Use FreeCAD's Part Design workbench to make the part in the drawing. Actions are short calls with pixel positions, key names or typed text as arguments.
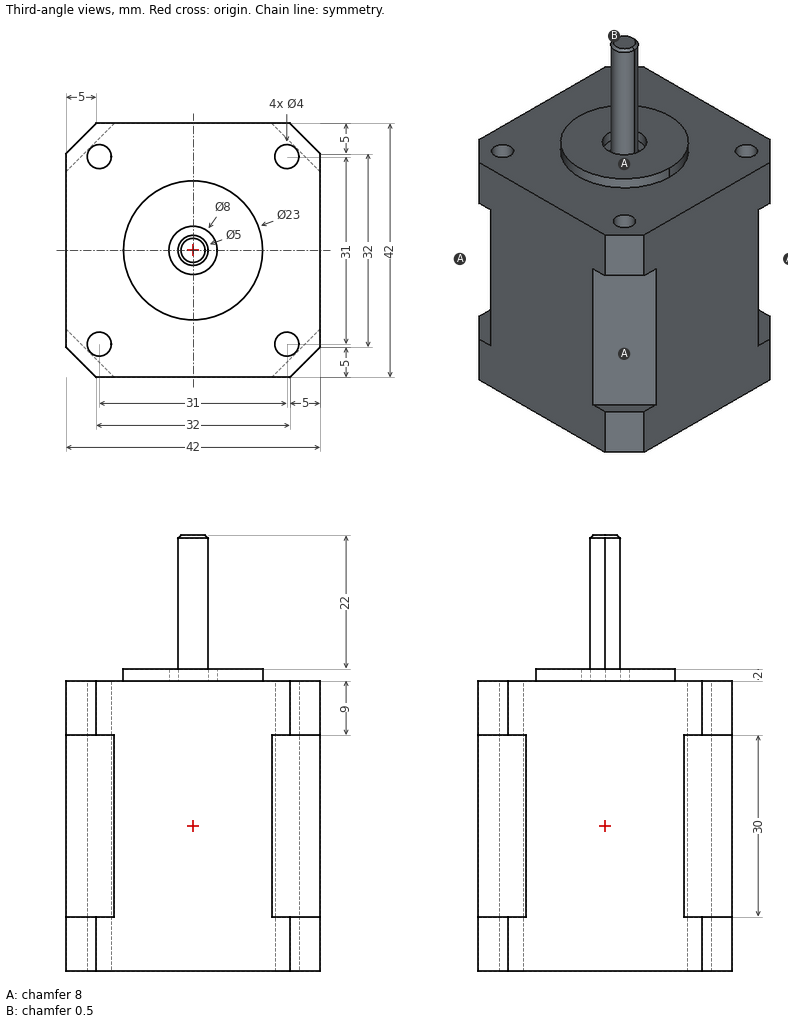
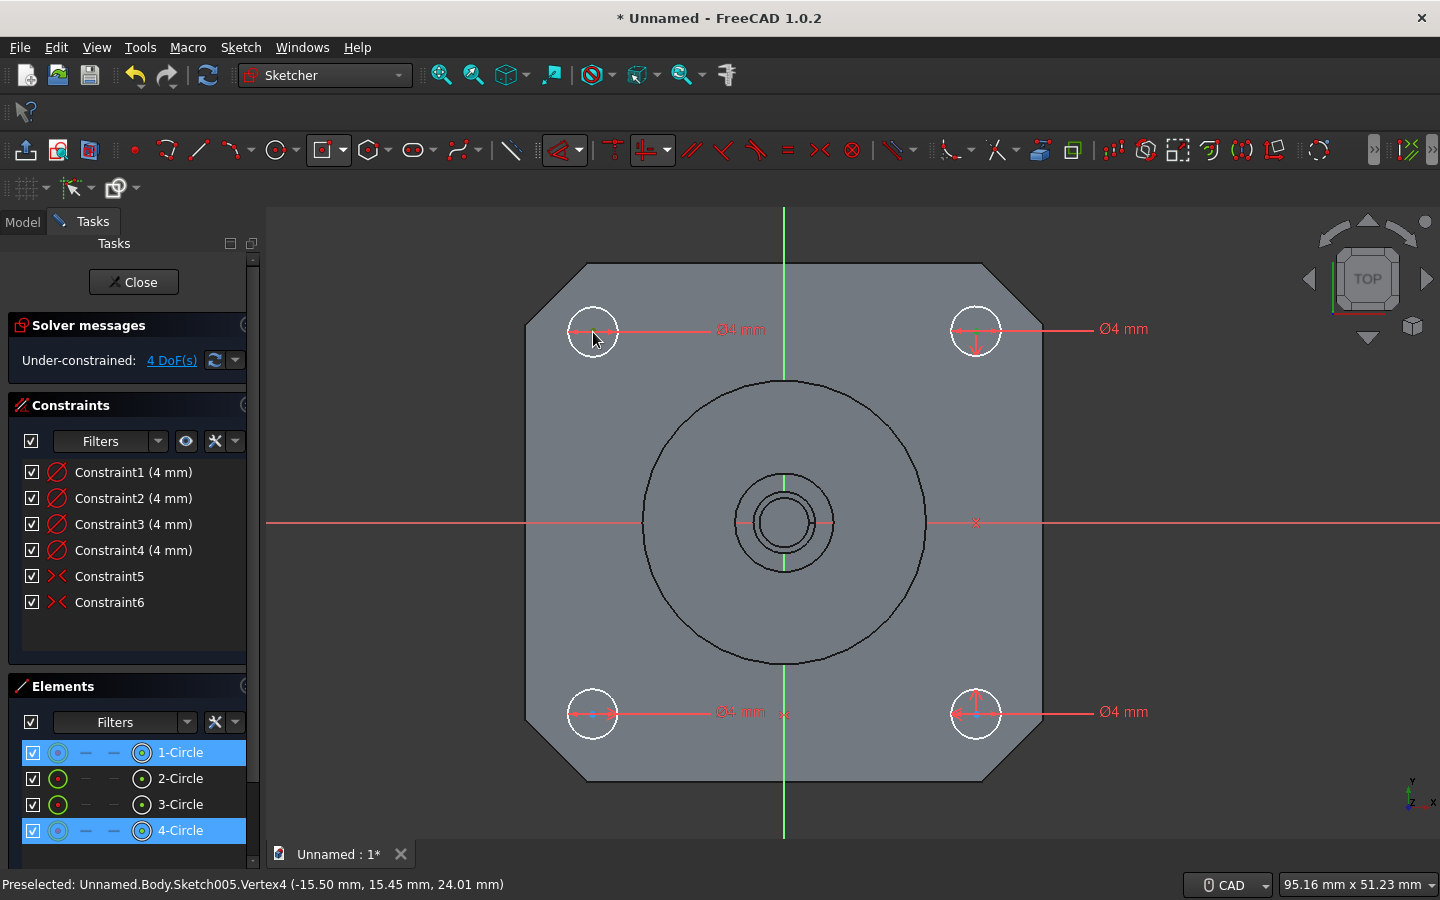
click(784, 770)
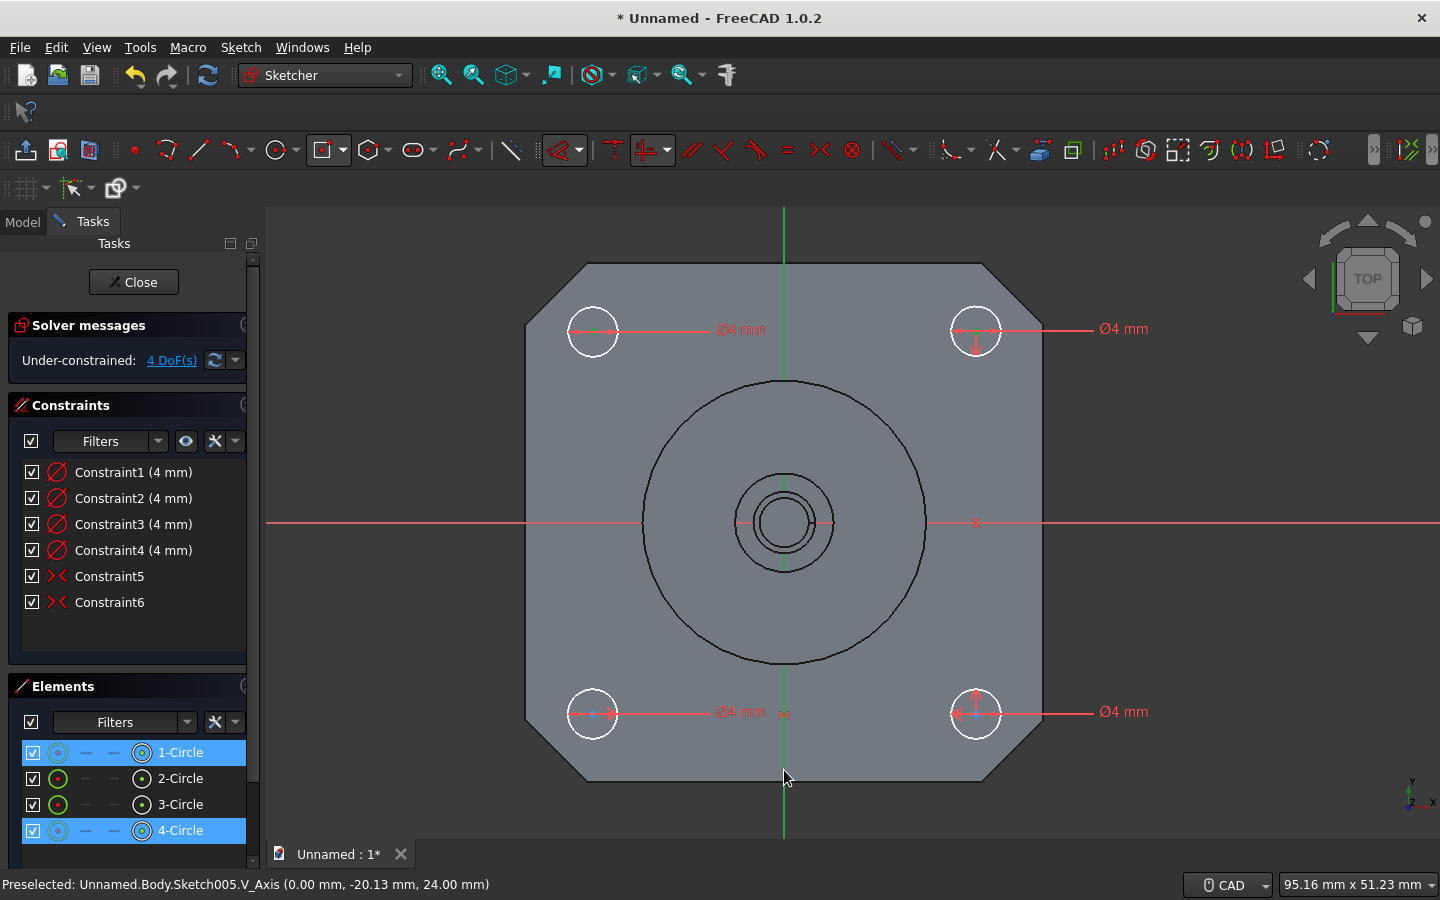
key(s)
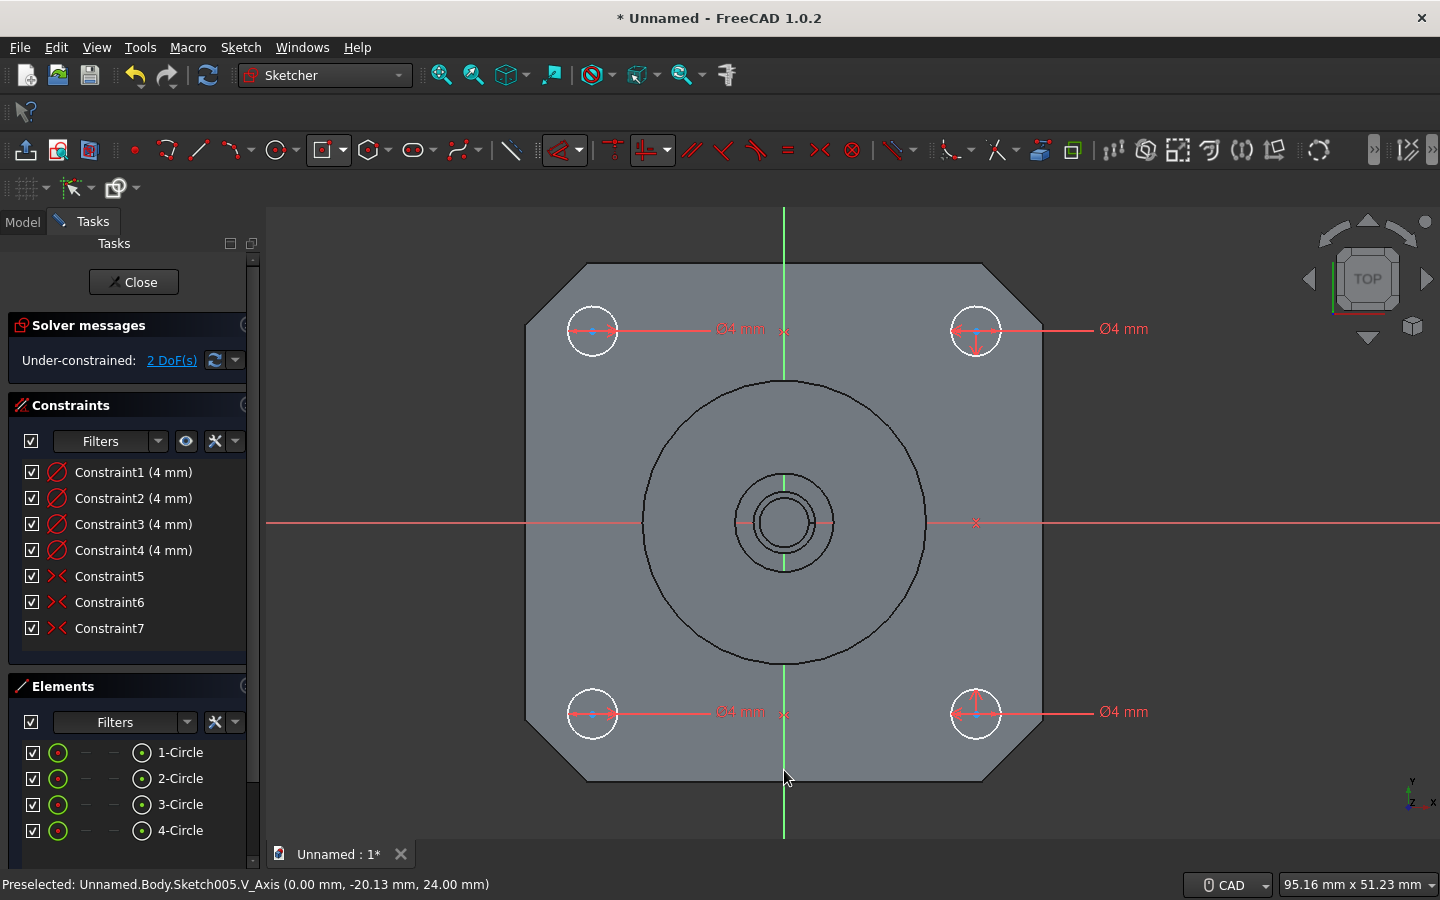
click(976, 331)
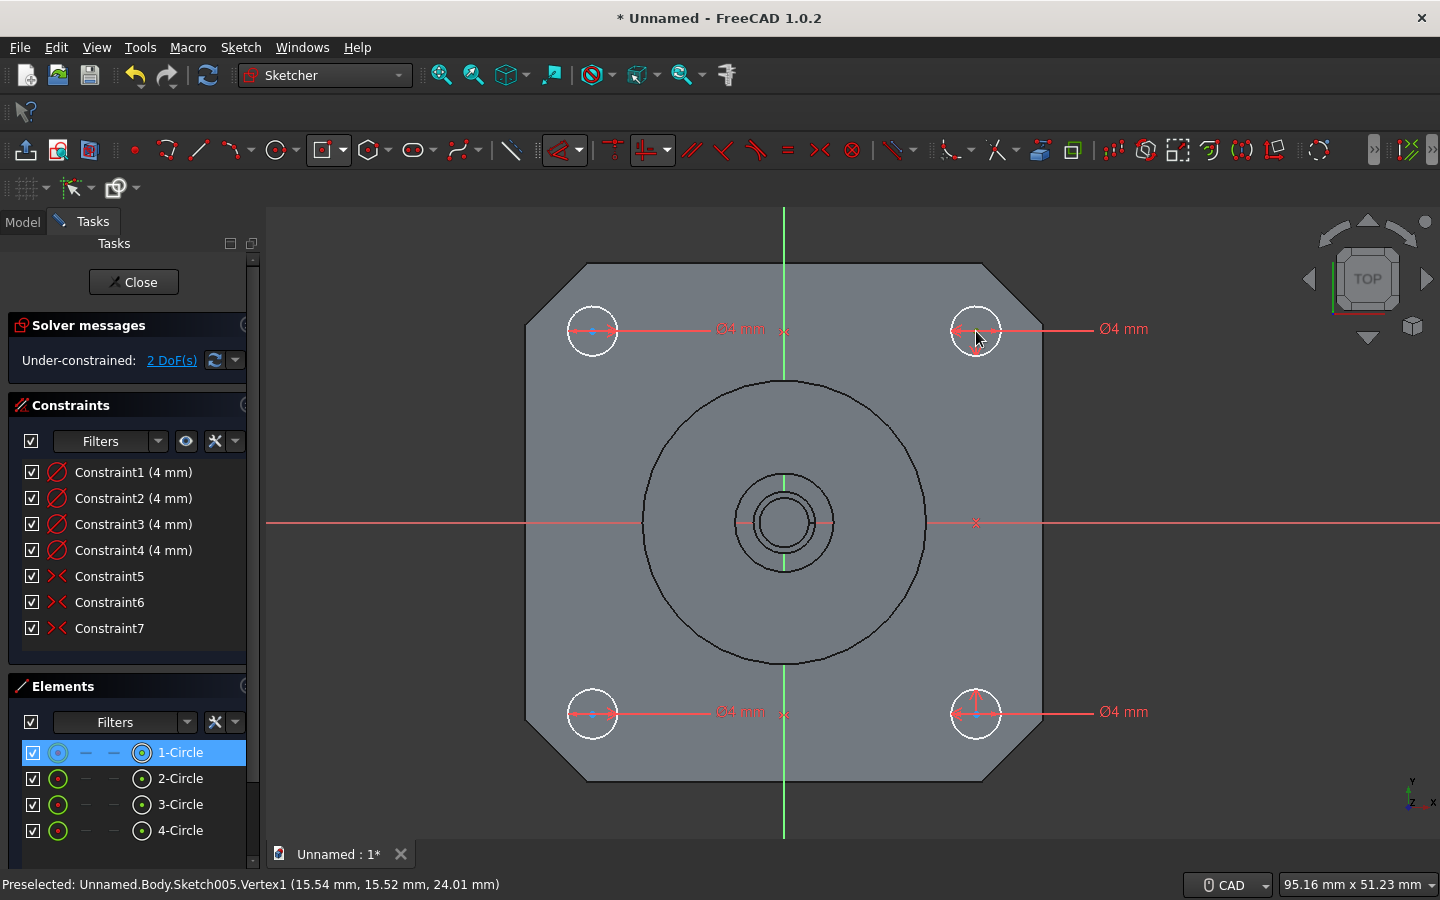
click(976, 714)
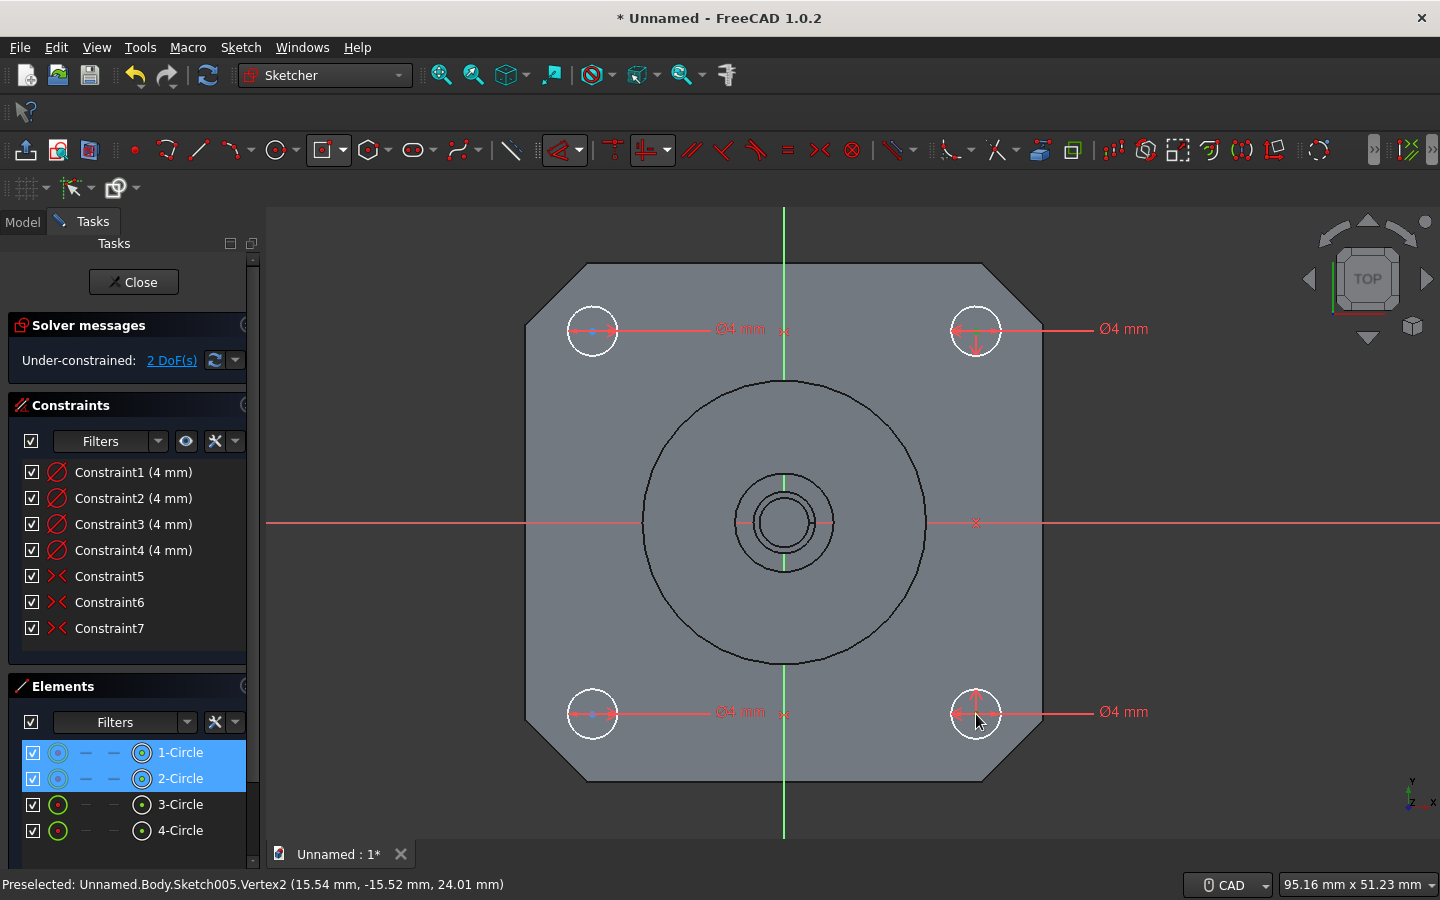
key(i)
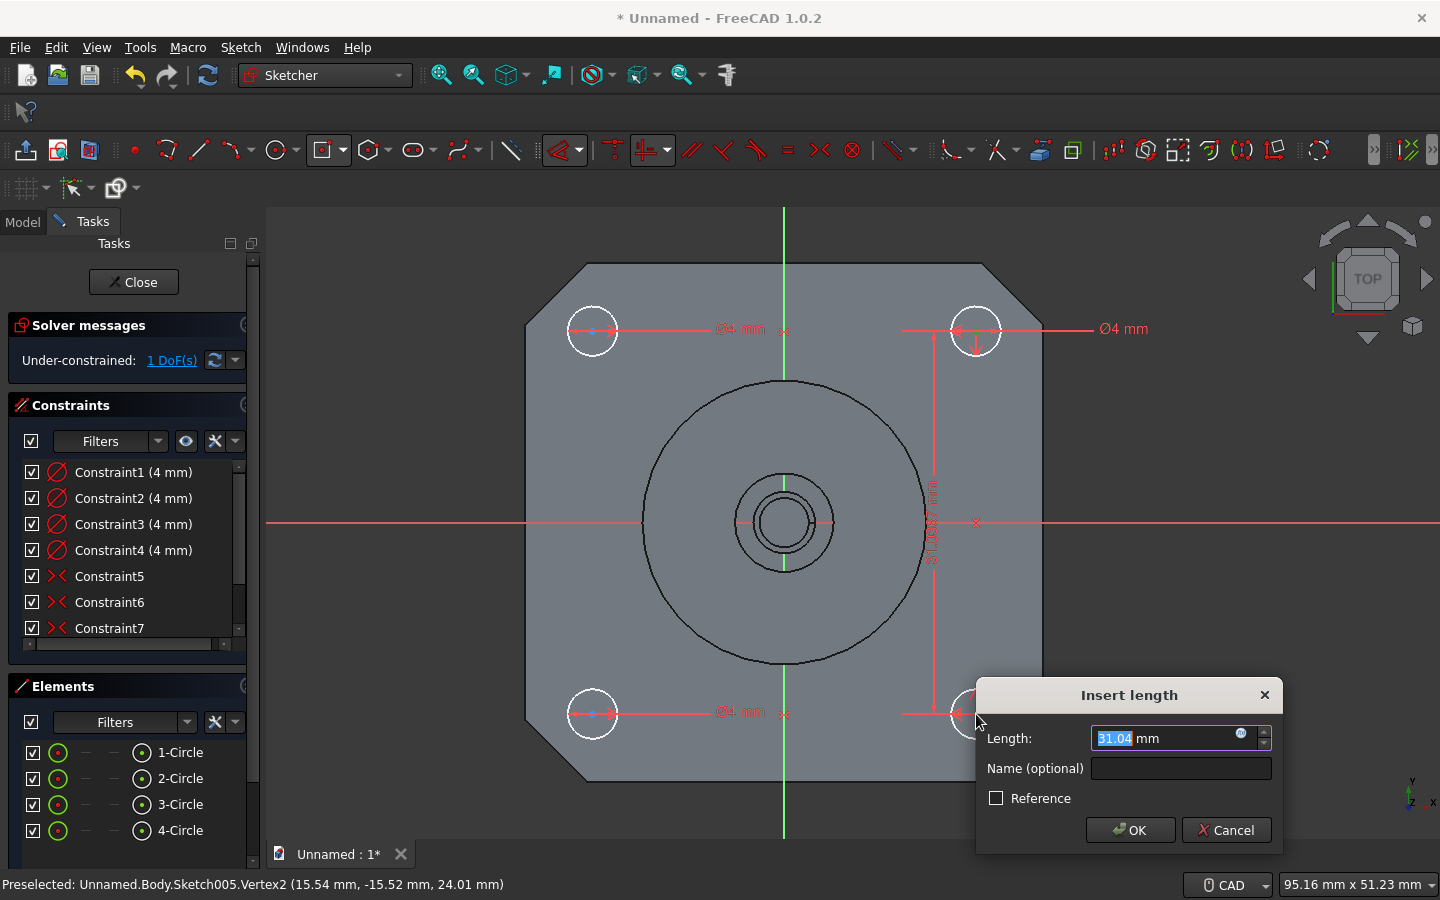
text(31)
key(Return)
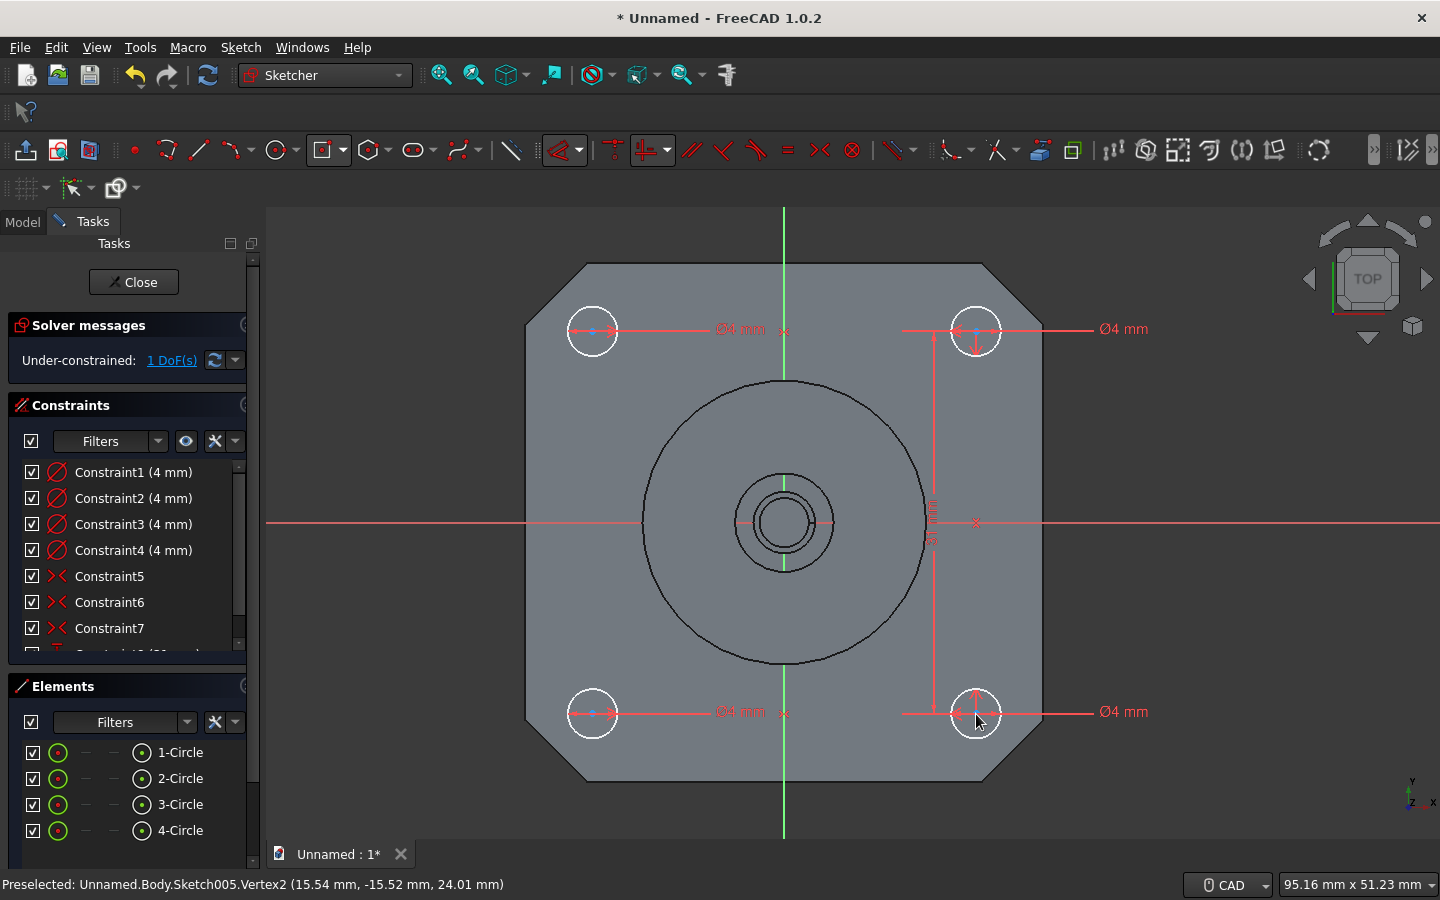
click(976, 714)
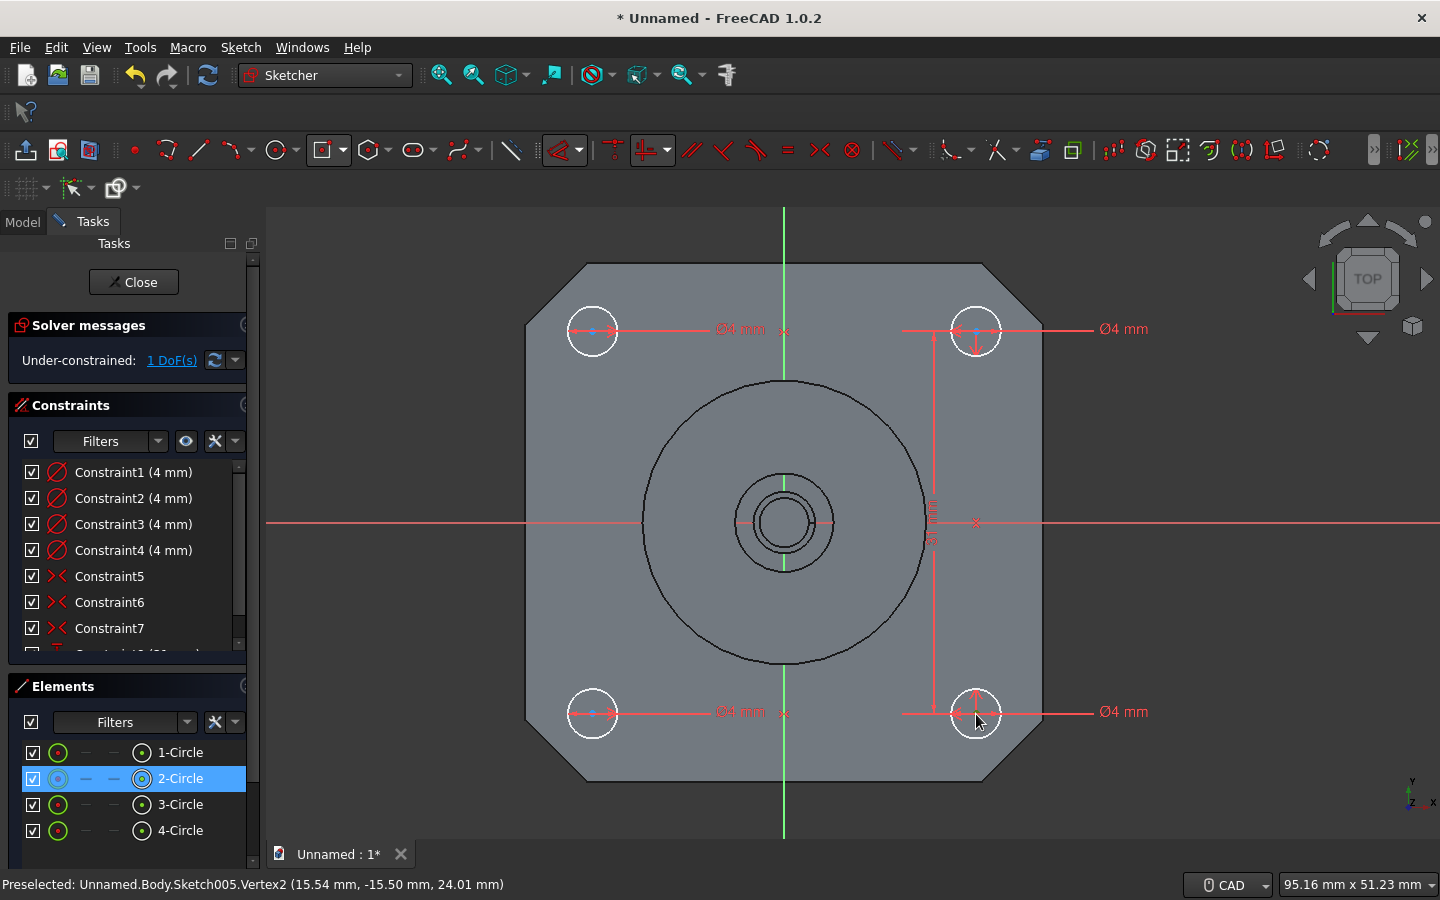
click(593, 714)